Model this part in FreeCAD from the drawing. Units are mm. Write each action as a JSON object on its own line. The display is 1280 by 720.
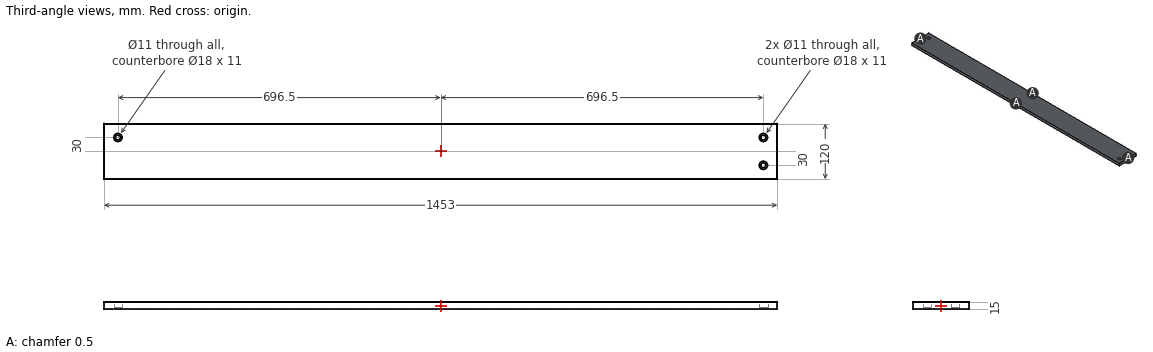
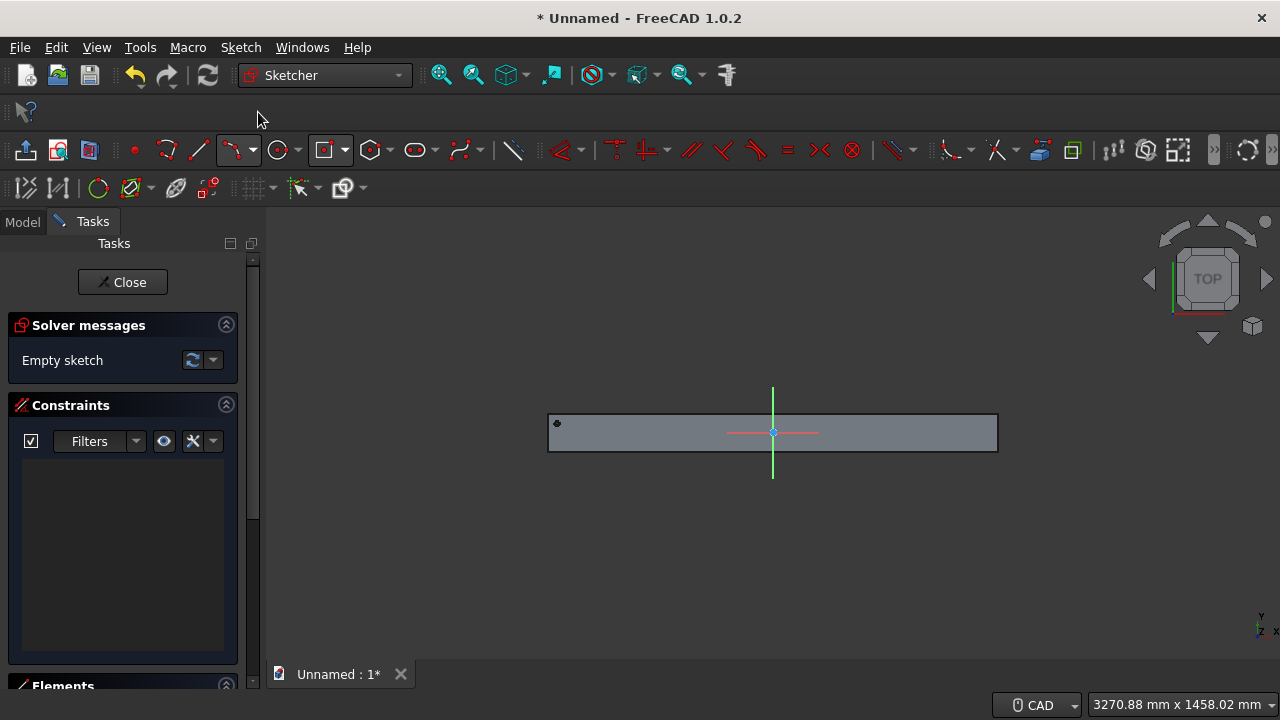
{"action": "scroll", "coordinate": [1012, 433], "scroll_direction": "up", "scroll_amount": 13}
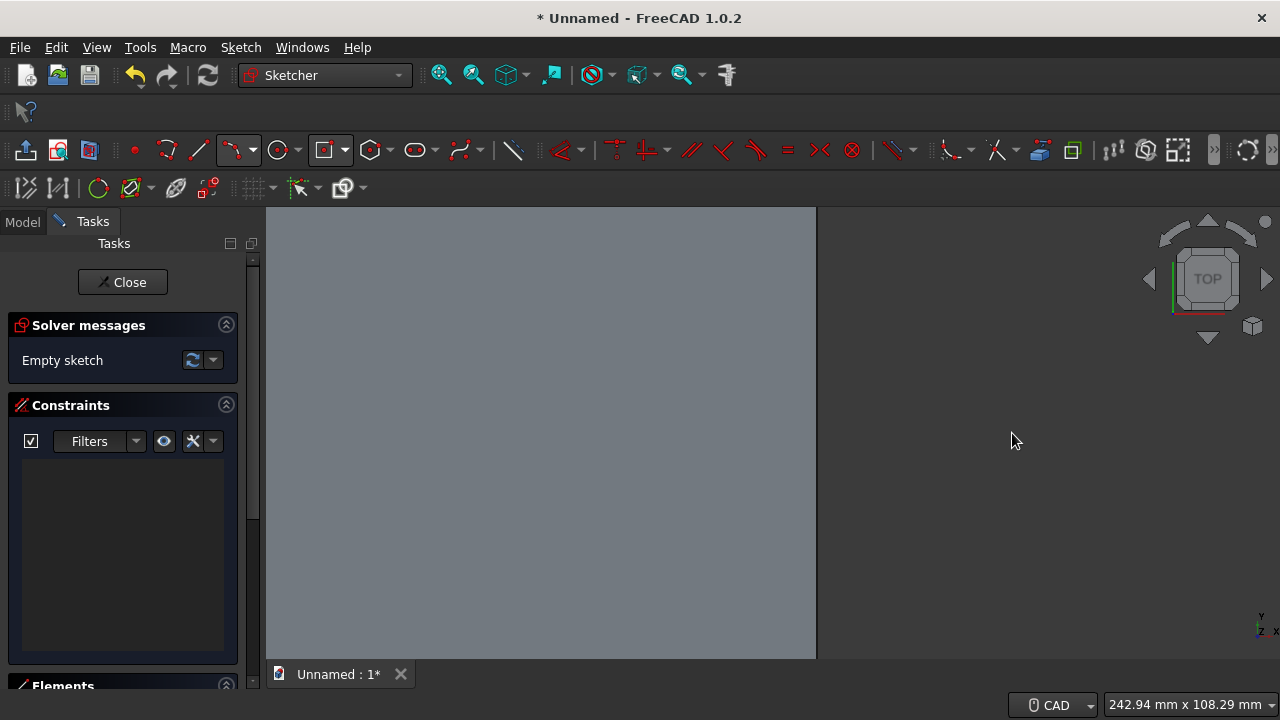
{"action": "key", "text": "g c"}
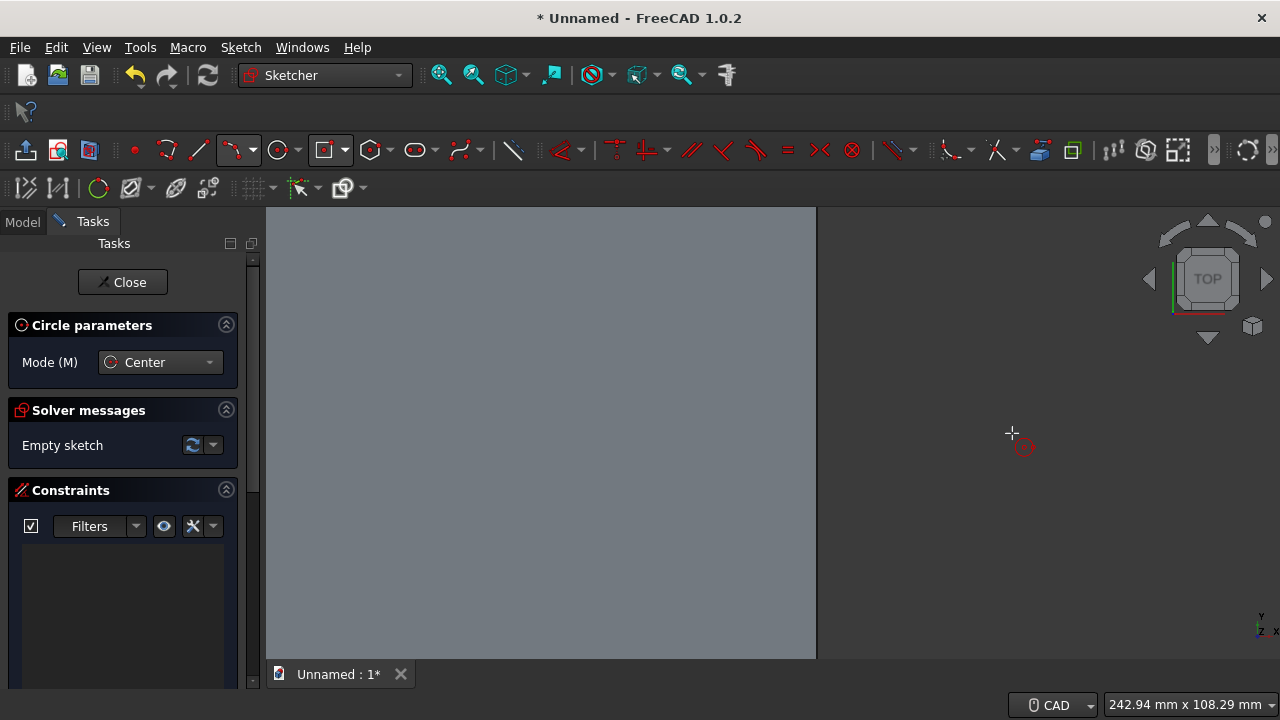
{"action": "left_click", "coordinate": [692, 302]}
{"action": "mouse_move", "coordinate": [708, 285]}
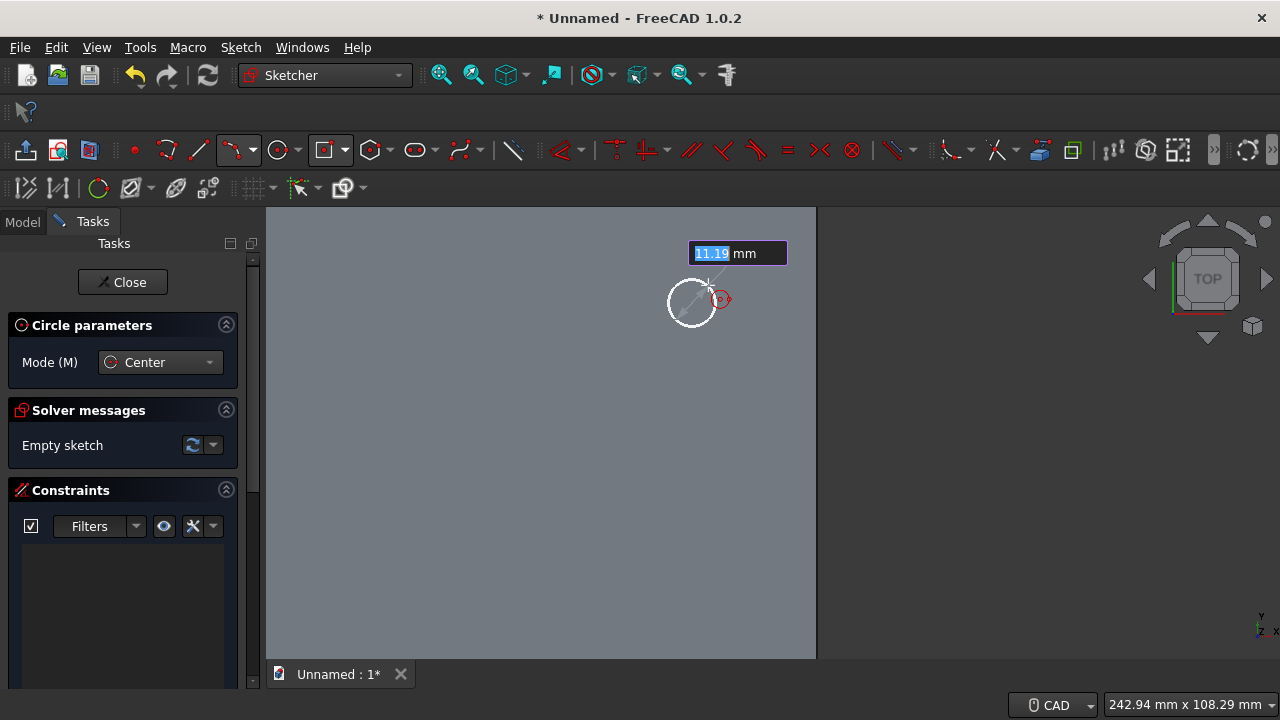
{"action": "type", "text": "11"}
{"action": "key", "text": "Return"}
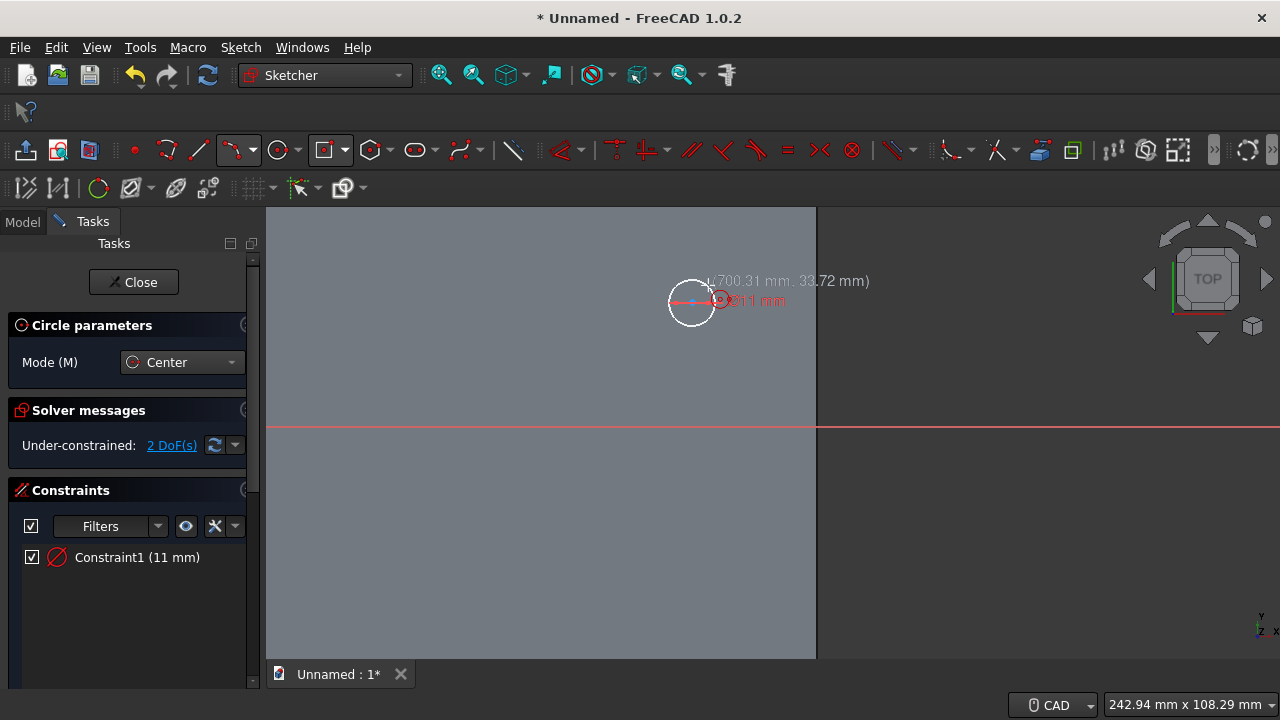
{"action": "left_click", "coordinate": [692, 552]}
{"action": "mouse_move", "coordinate": [708, 536]}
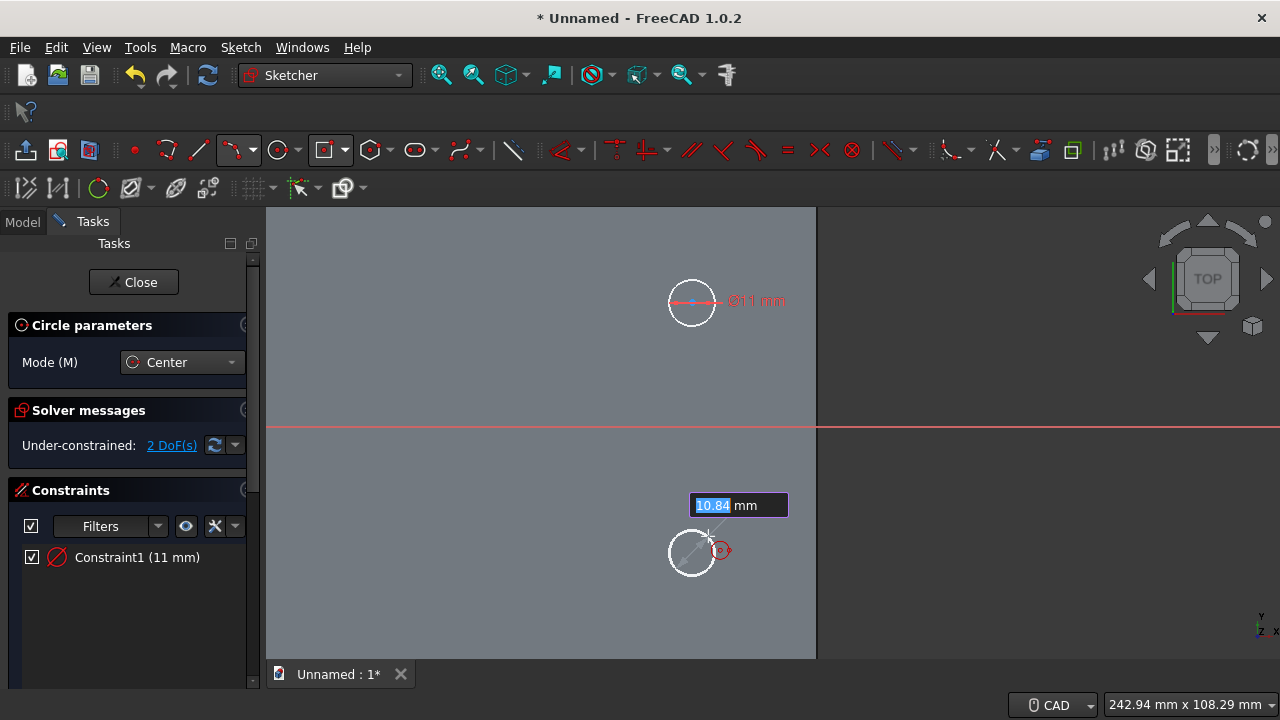
{"action": "type", "text": "11"}
{"action": "key", "text": "Return"}
{"action": "key", "text": "Escape"}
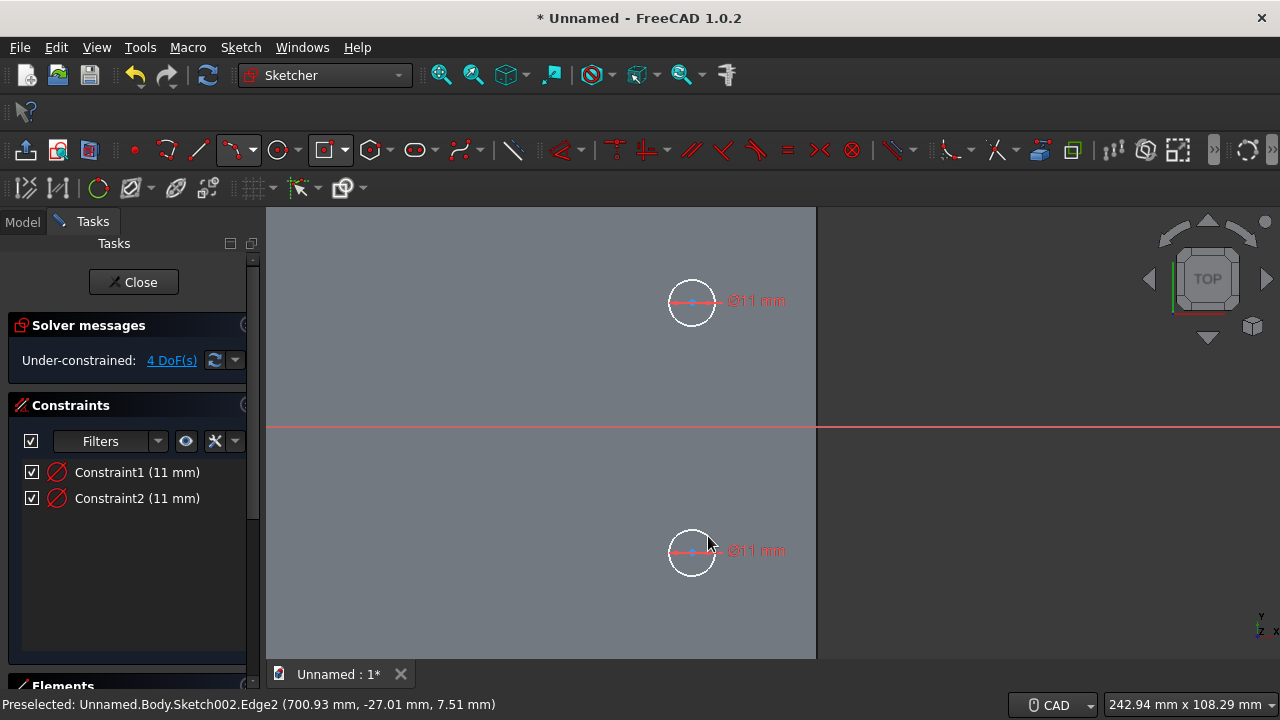
{"action": "left_click", "coordinate": [692, 303]}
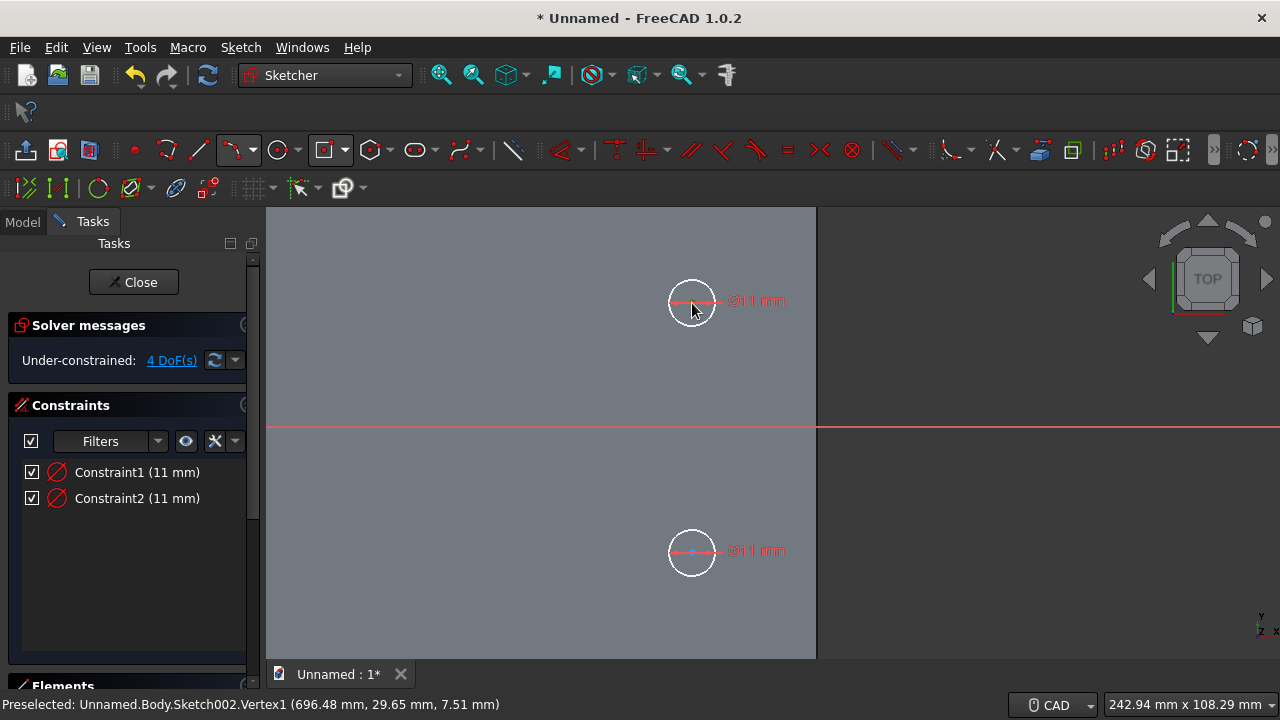
{"action": "left_click", "coordinate": [692, 553]}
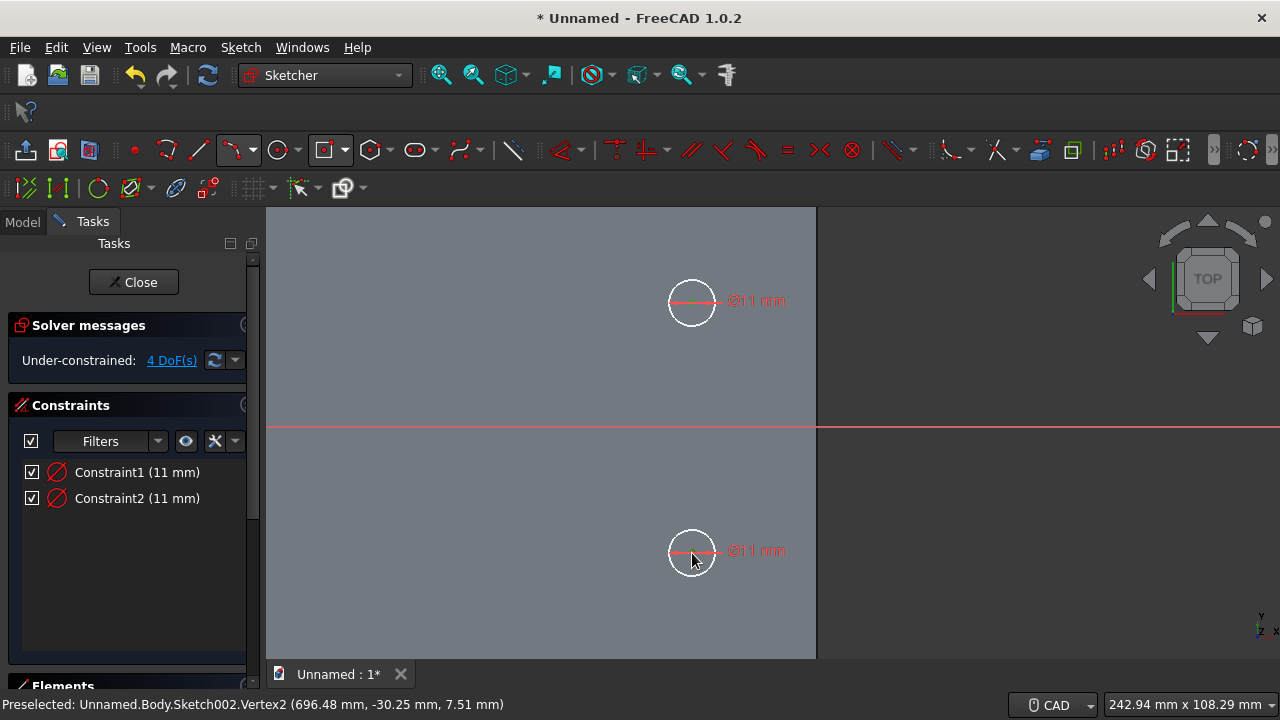
{"action": "left_click", "coordinate": [670, 150]}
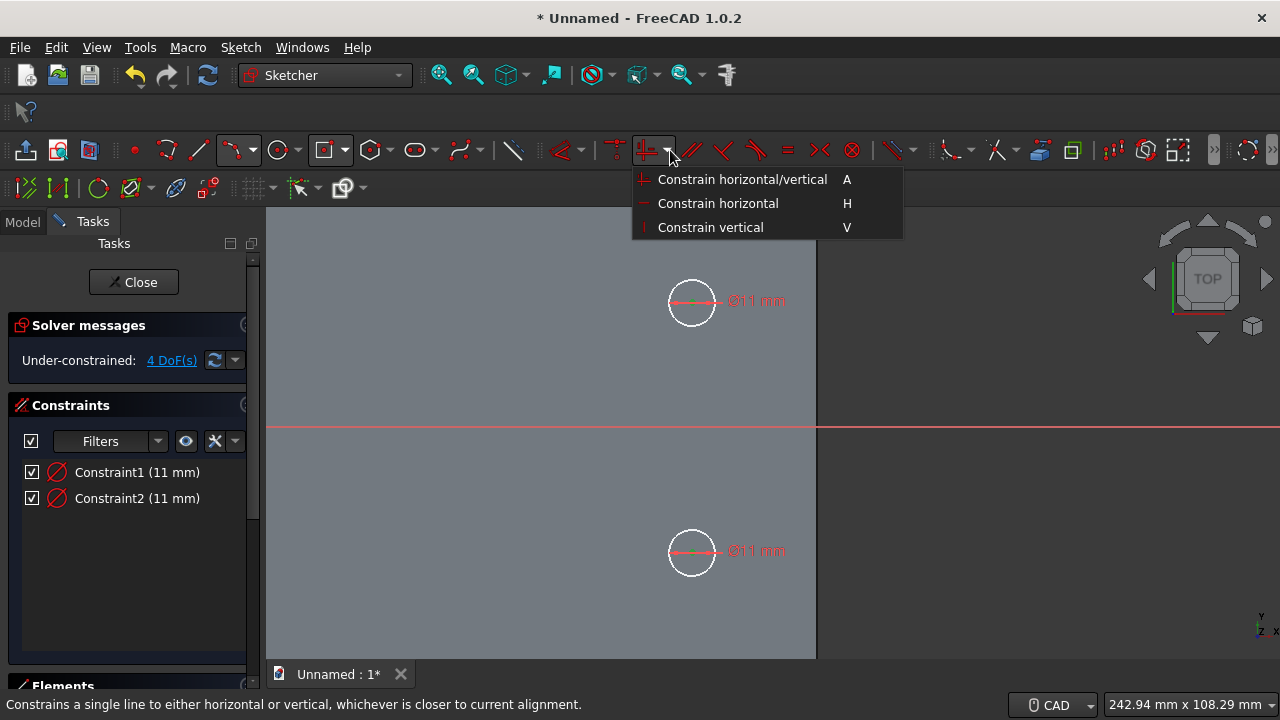
{"action": "left_click", "coordinate": [768, 227]}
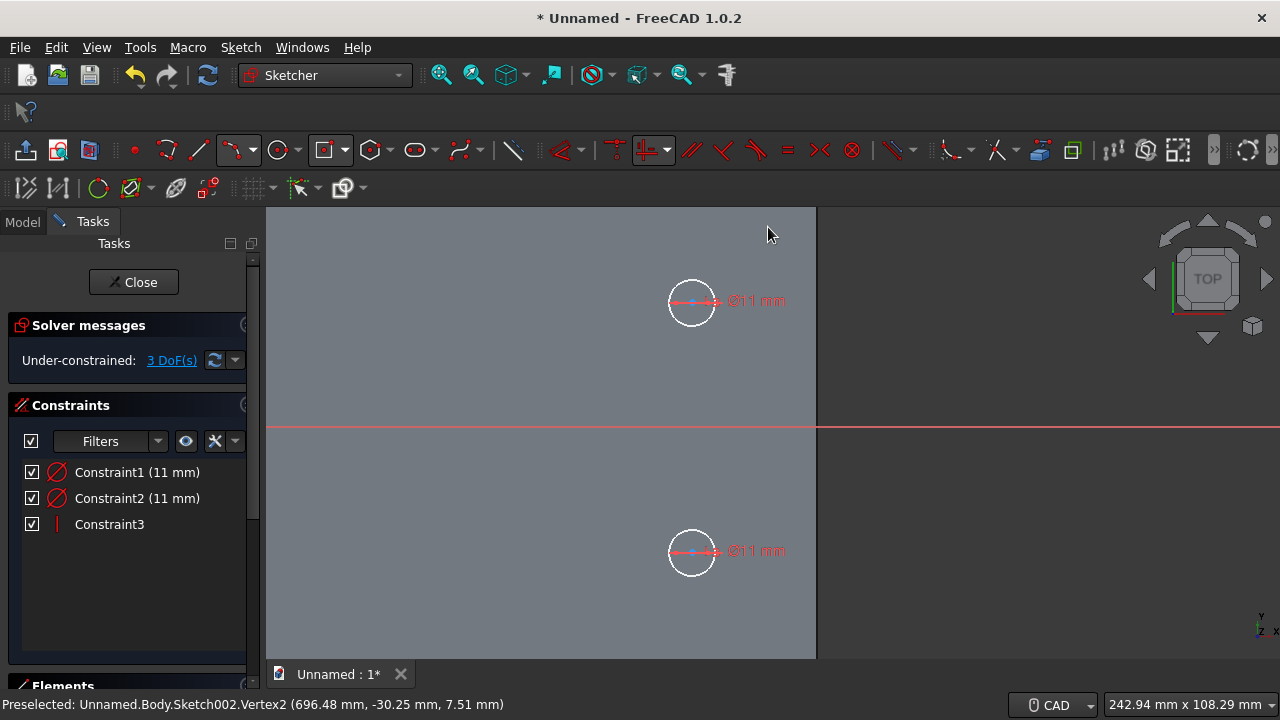
{"action": "left_click", "coordinate": [560, 150]}